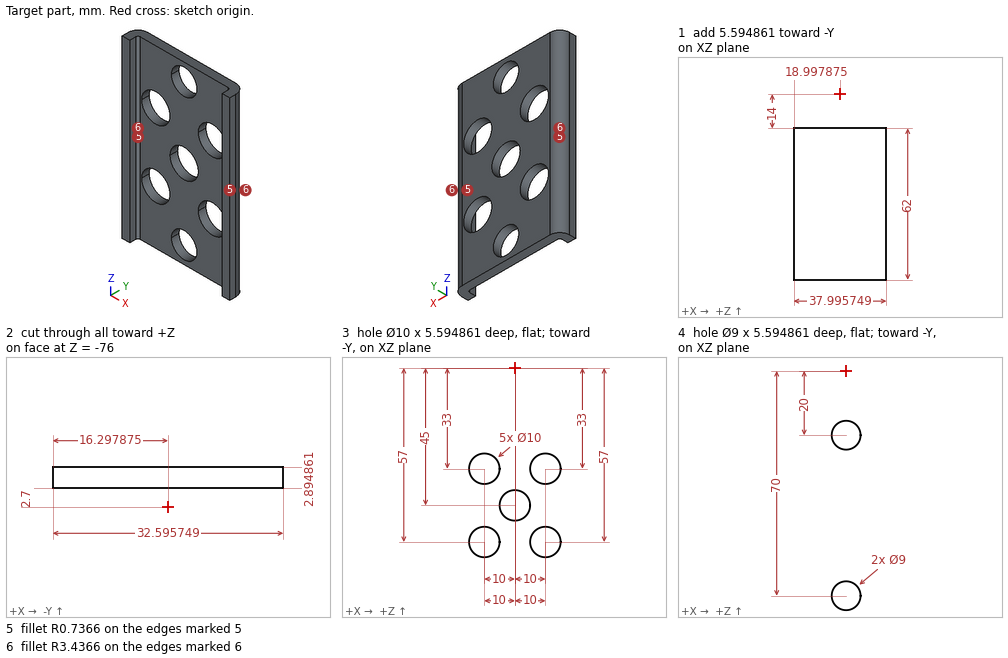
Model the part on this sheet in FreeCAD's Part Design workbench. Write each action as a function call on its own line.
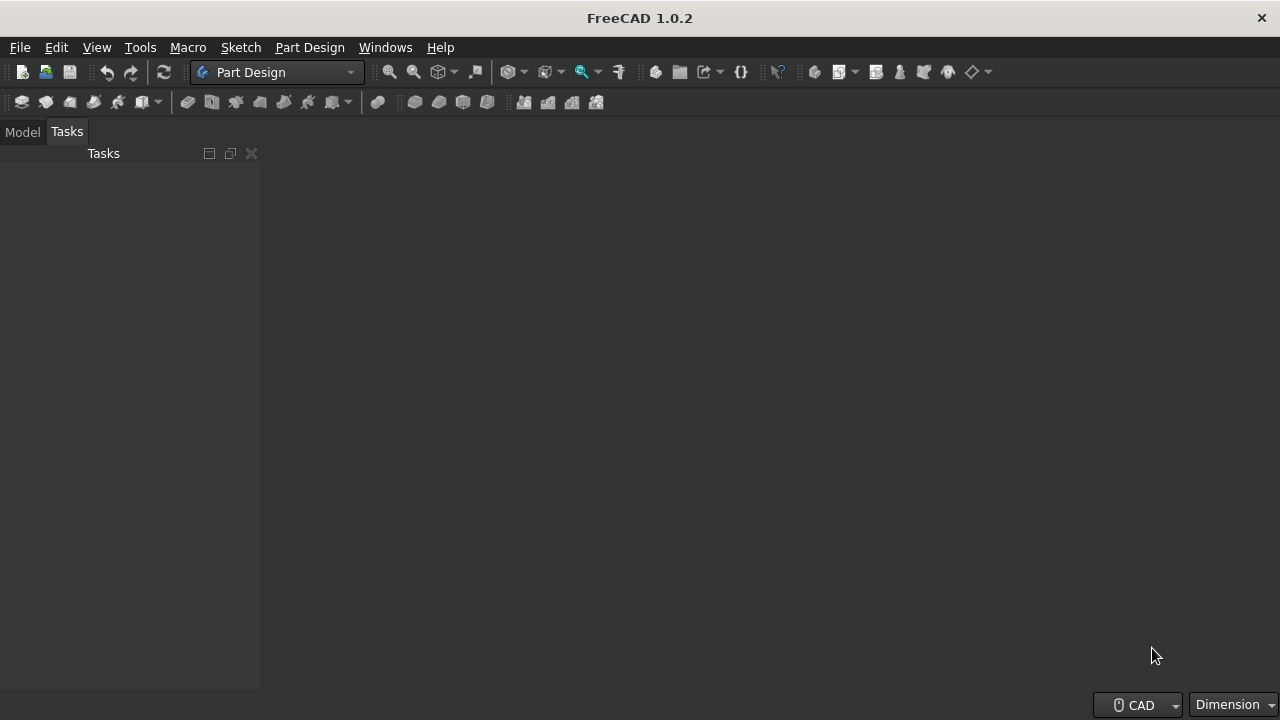
key(ctrl+n)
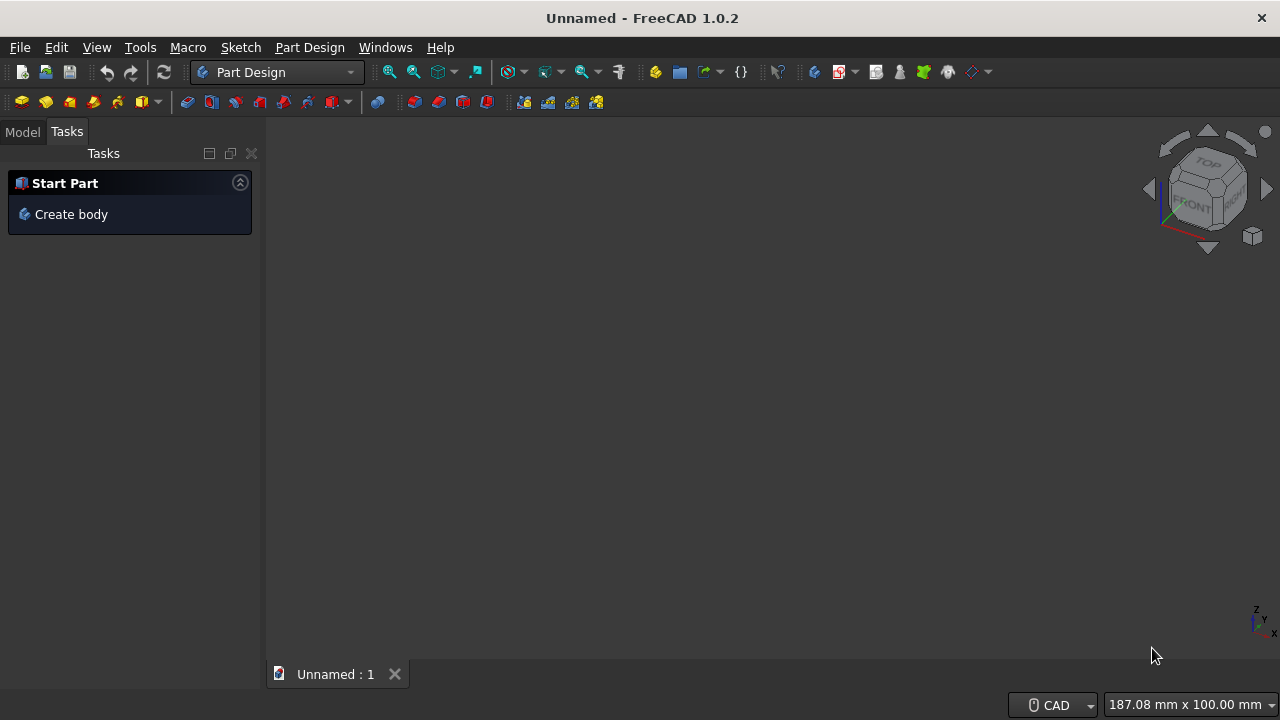
click(840, 72)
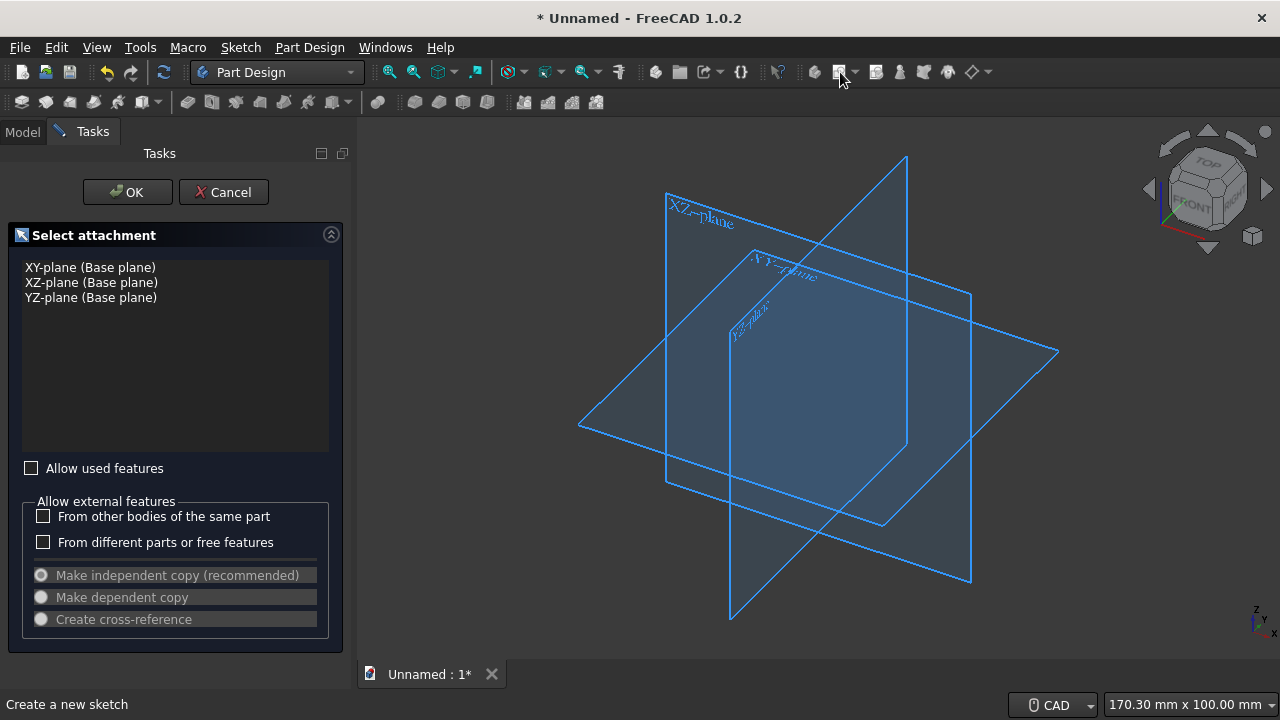
click(82, 282)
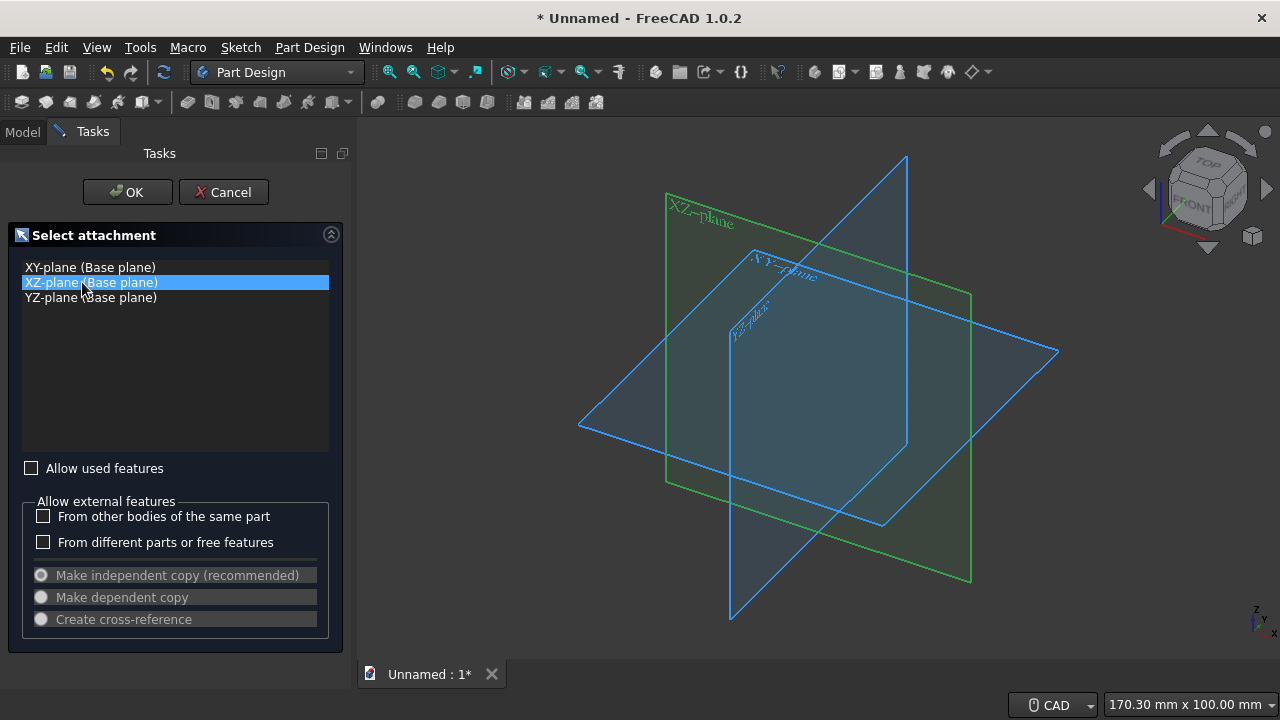
click(128, 192)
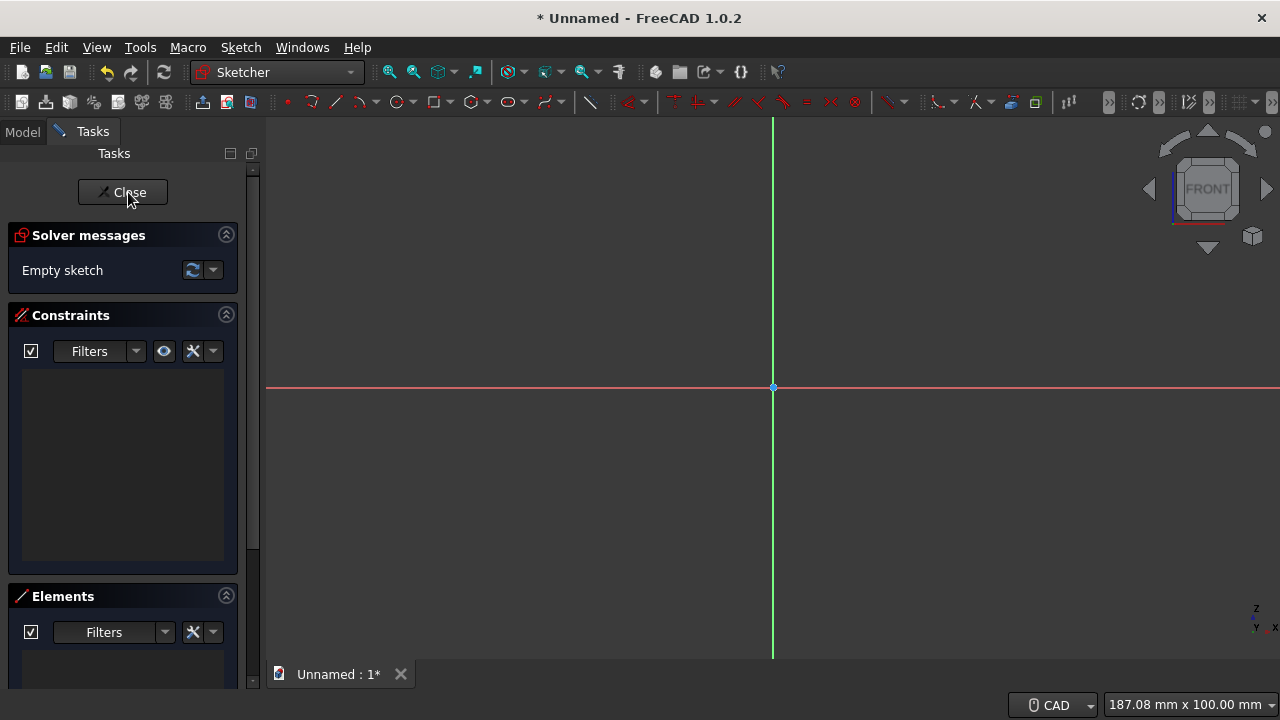
scroll(565, 145, down, 2)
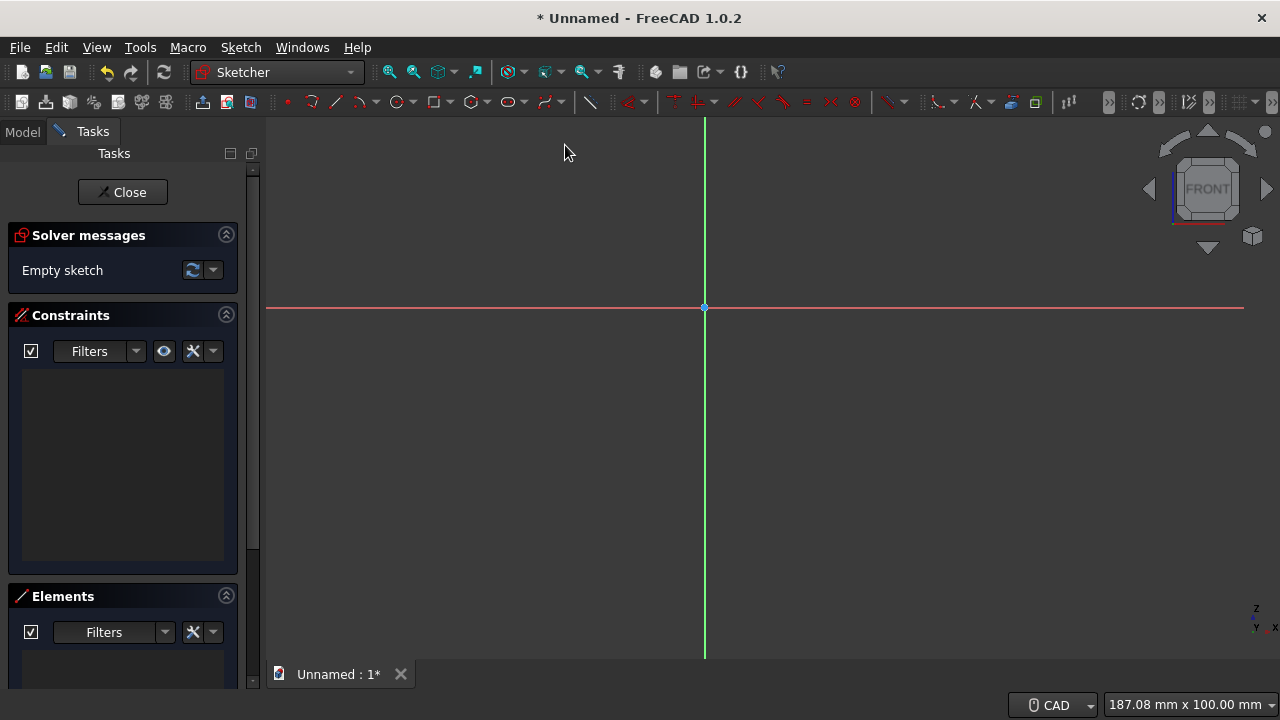
key(g)
key(r)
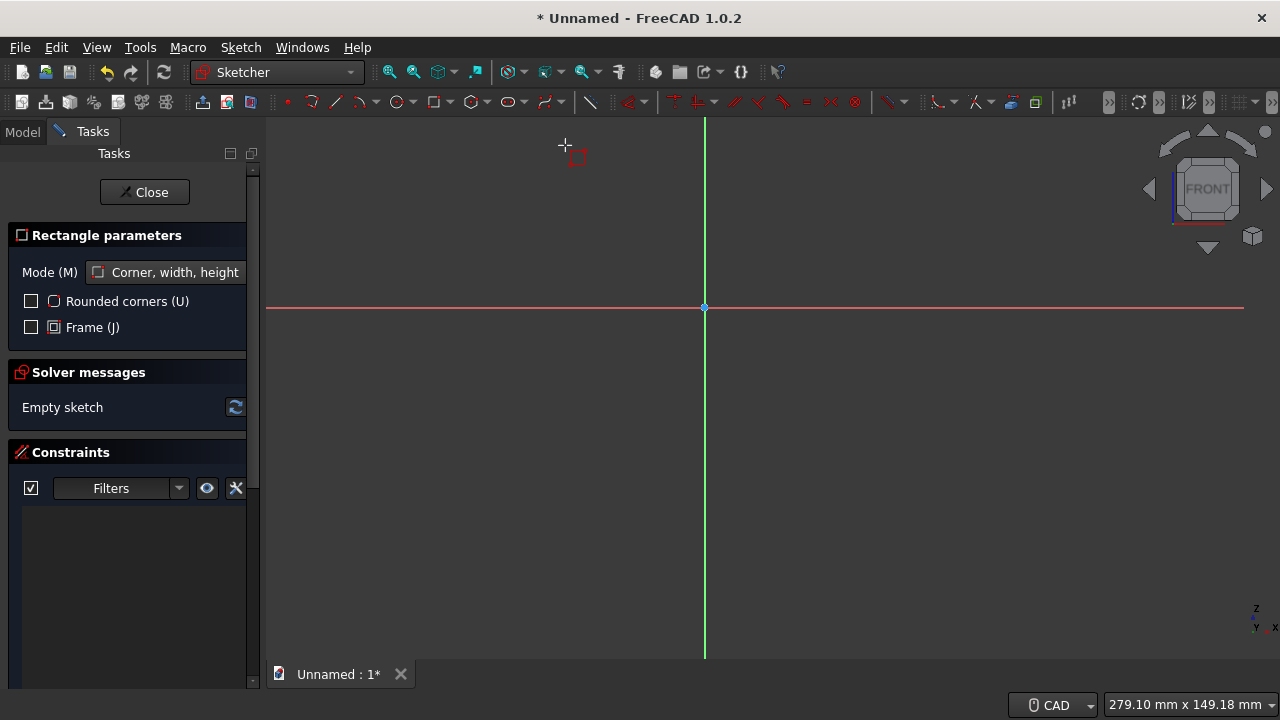
click(636, 359)
move(774, 584)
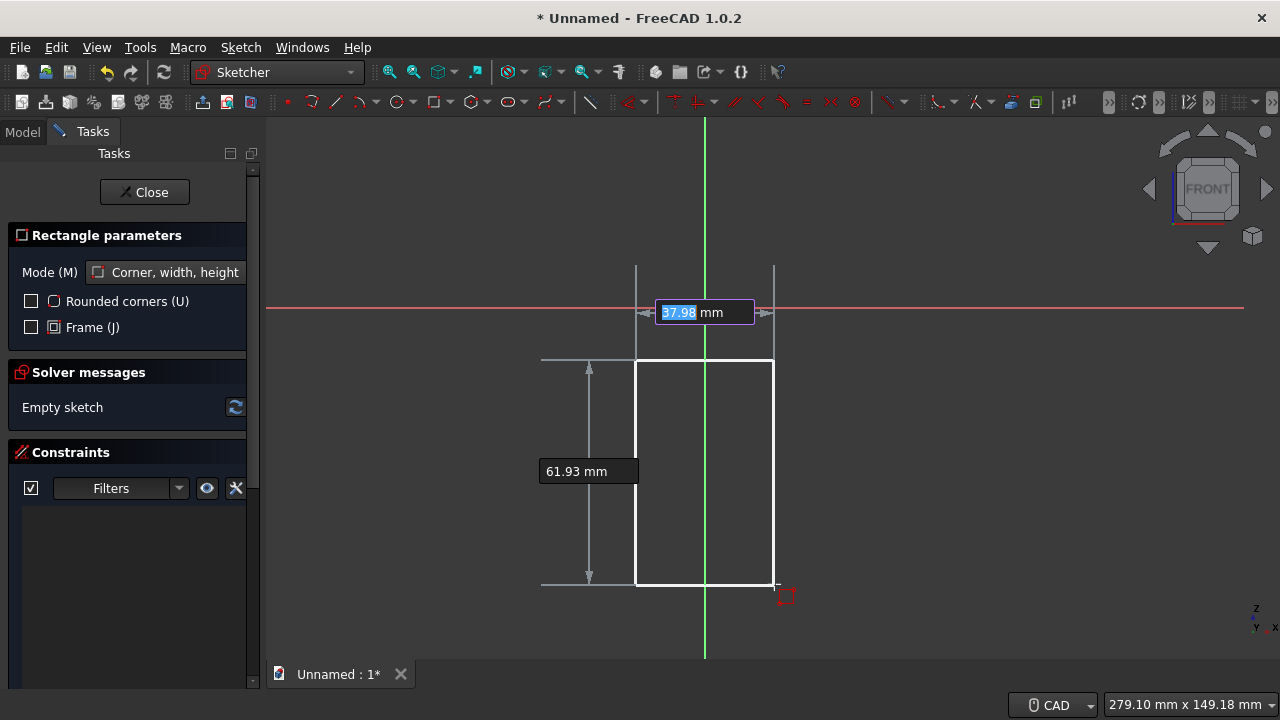
text(37.995749)
key(Tab)
text(62)
key(Return)
key(Escape)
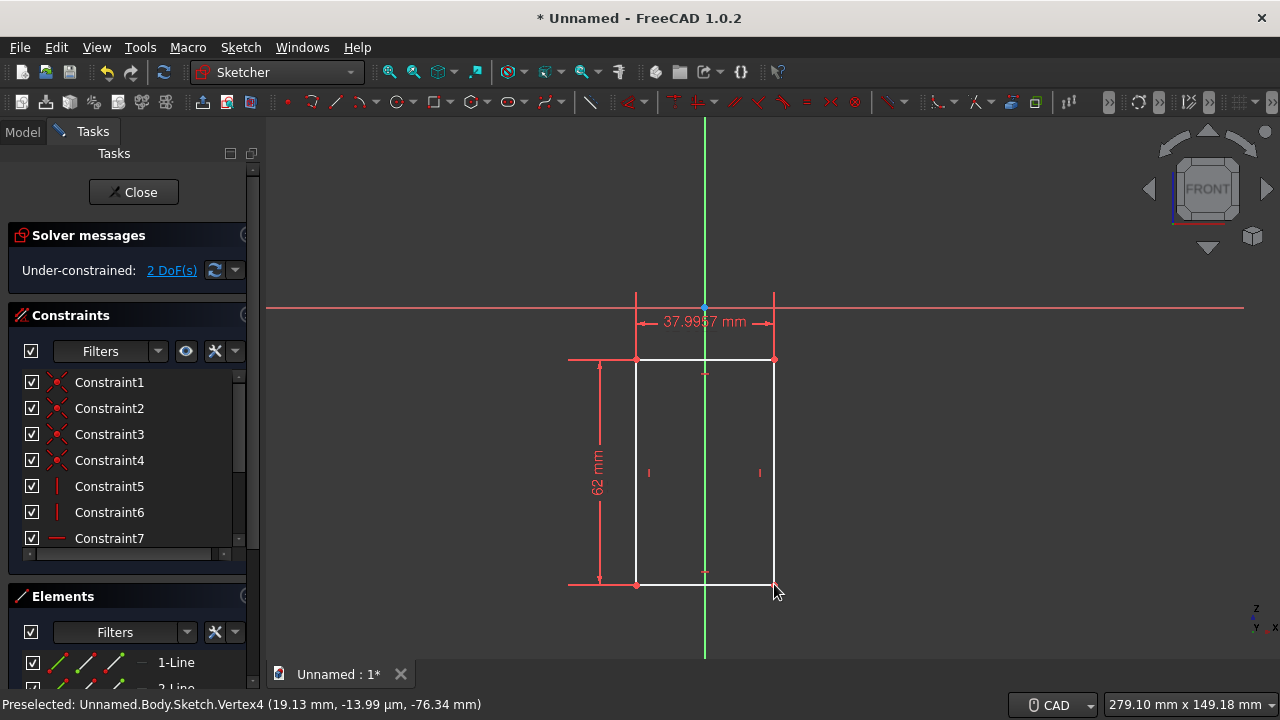
key(d)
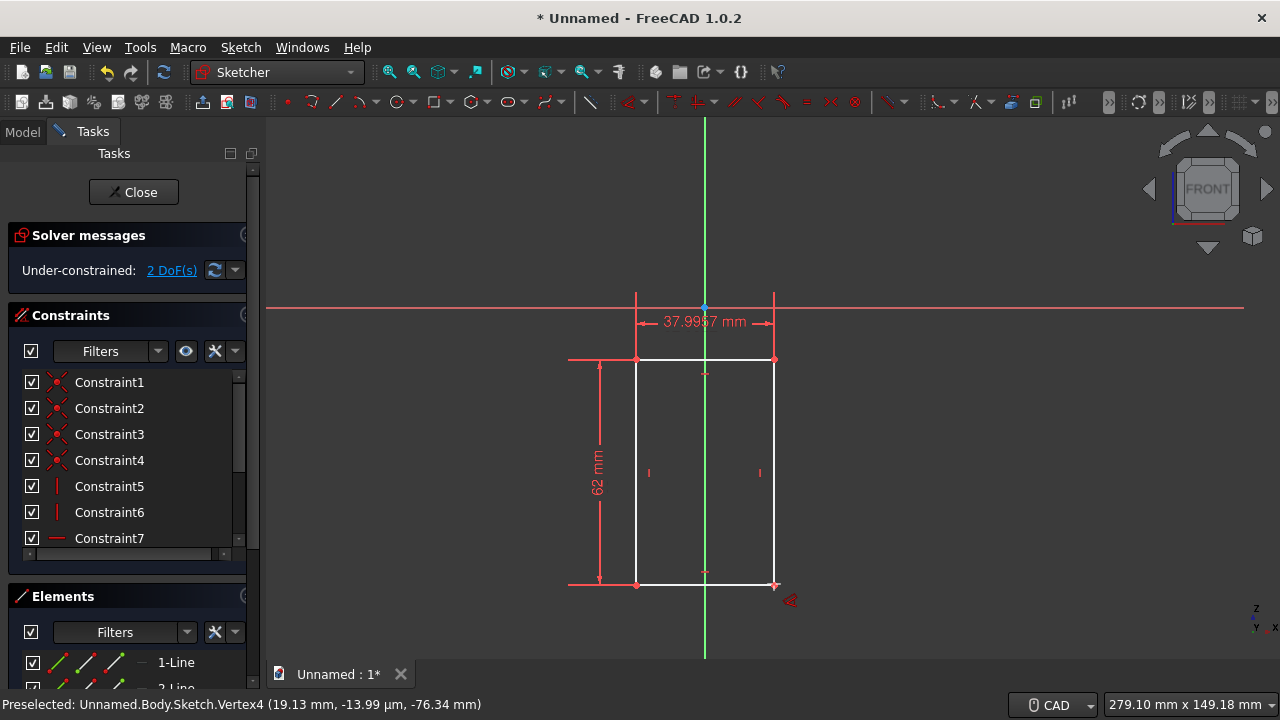
click(636, 360)
click(602, 334)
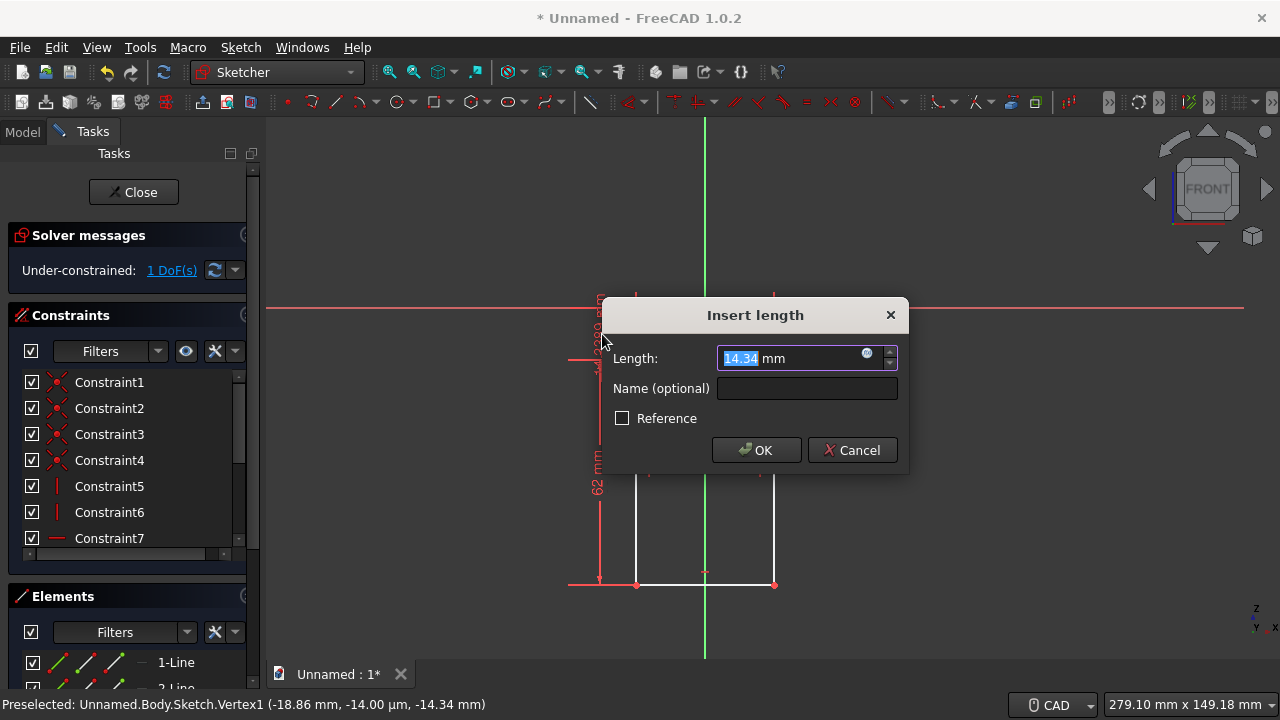
text(14)
key(Return)